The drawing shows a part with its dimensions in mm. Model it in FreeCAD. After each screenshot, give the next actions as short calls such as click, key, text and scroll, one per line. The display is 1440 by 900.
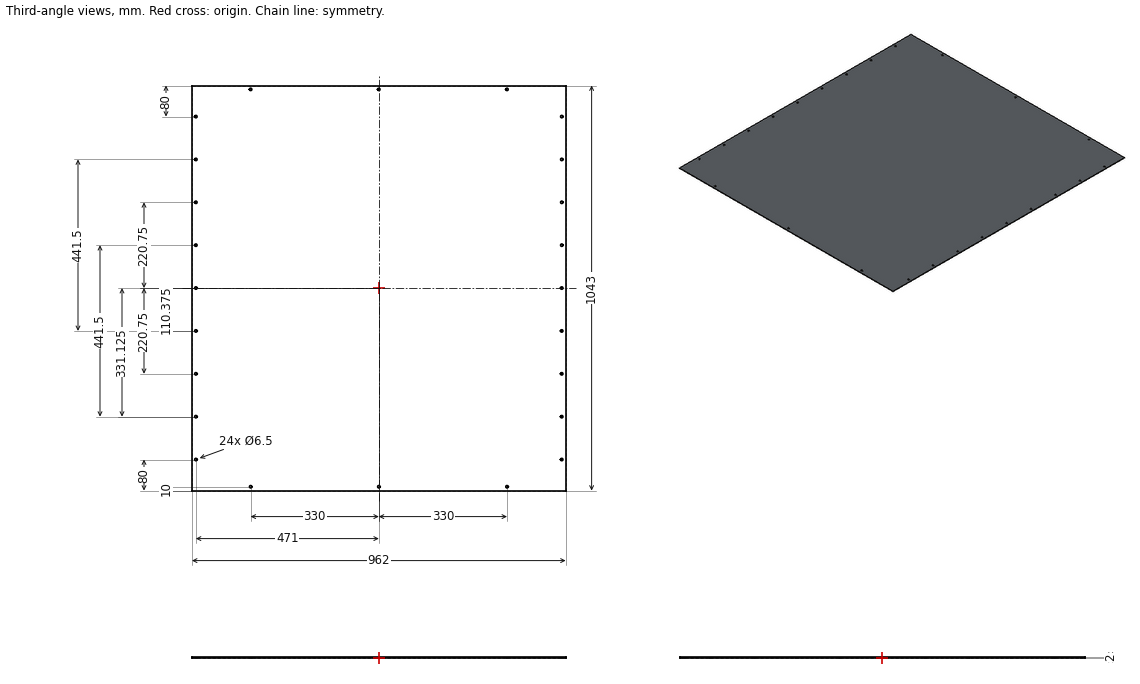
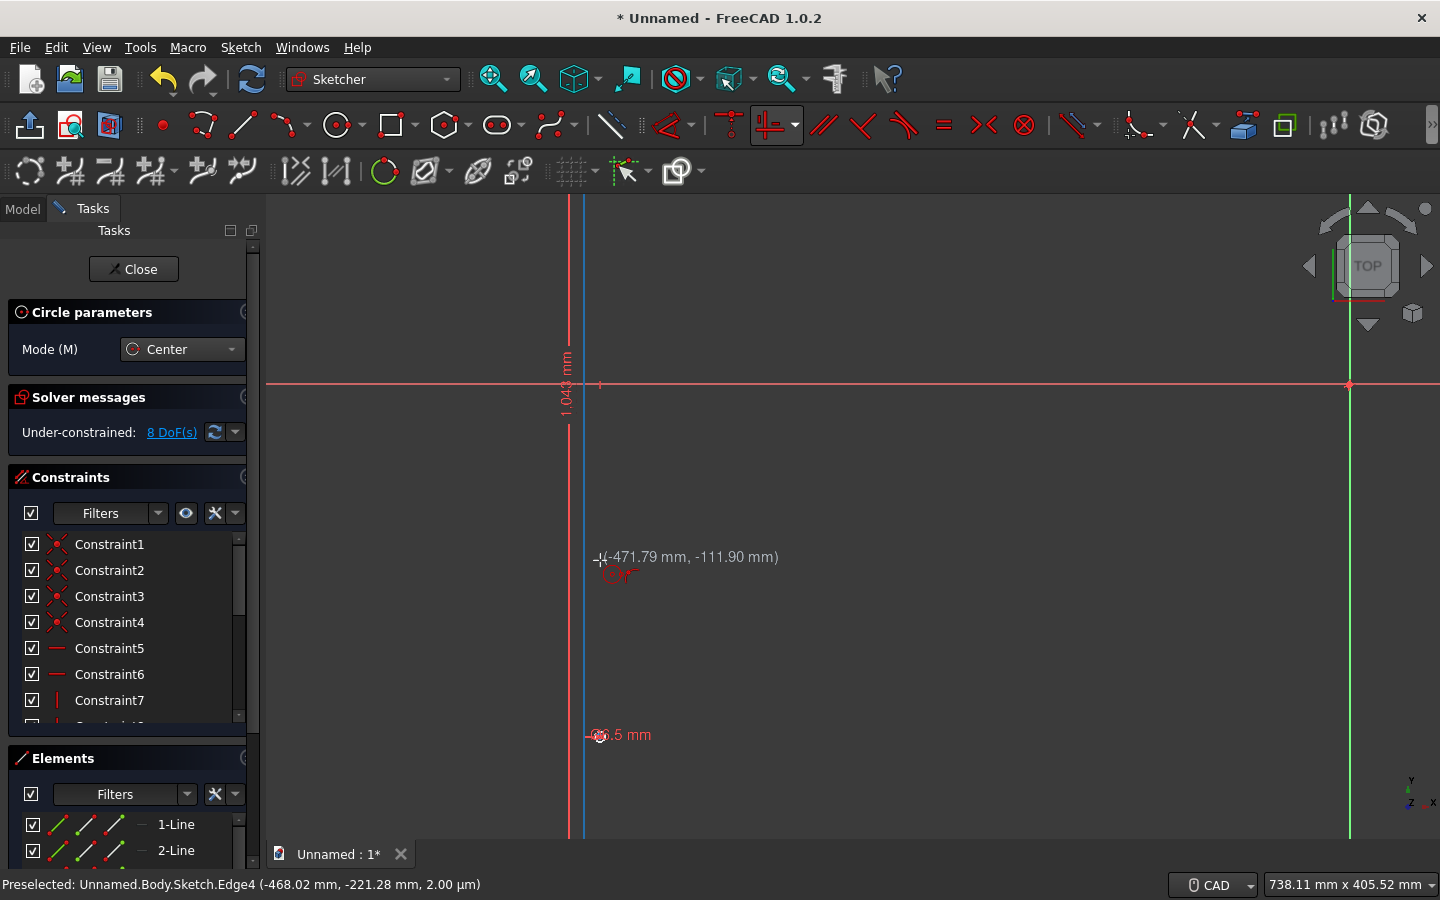
click(600, 560)
move(604, 556)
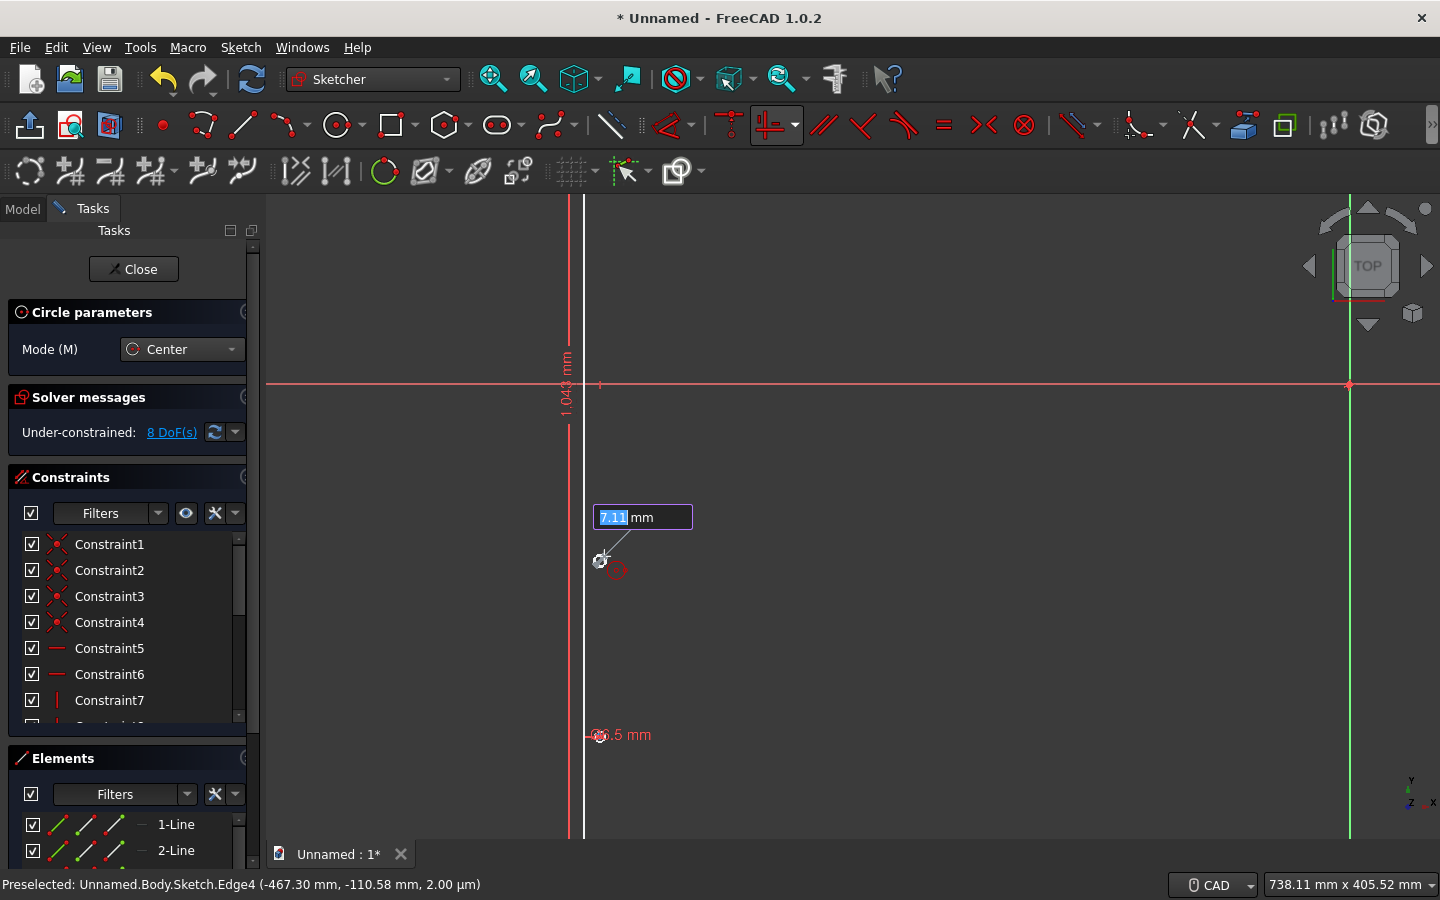
text(6.5)
key(Return)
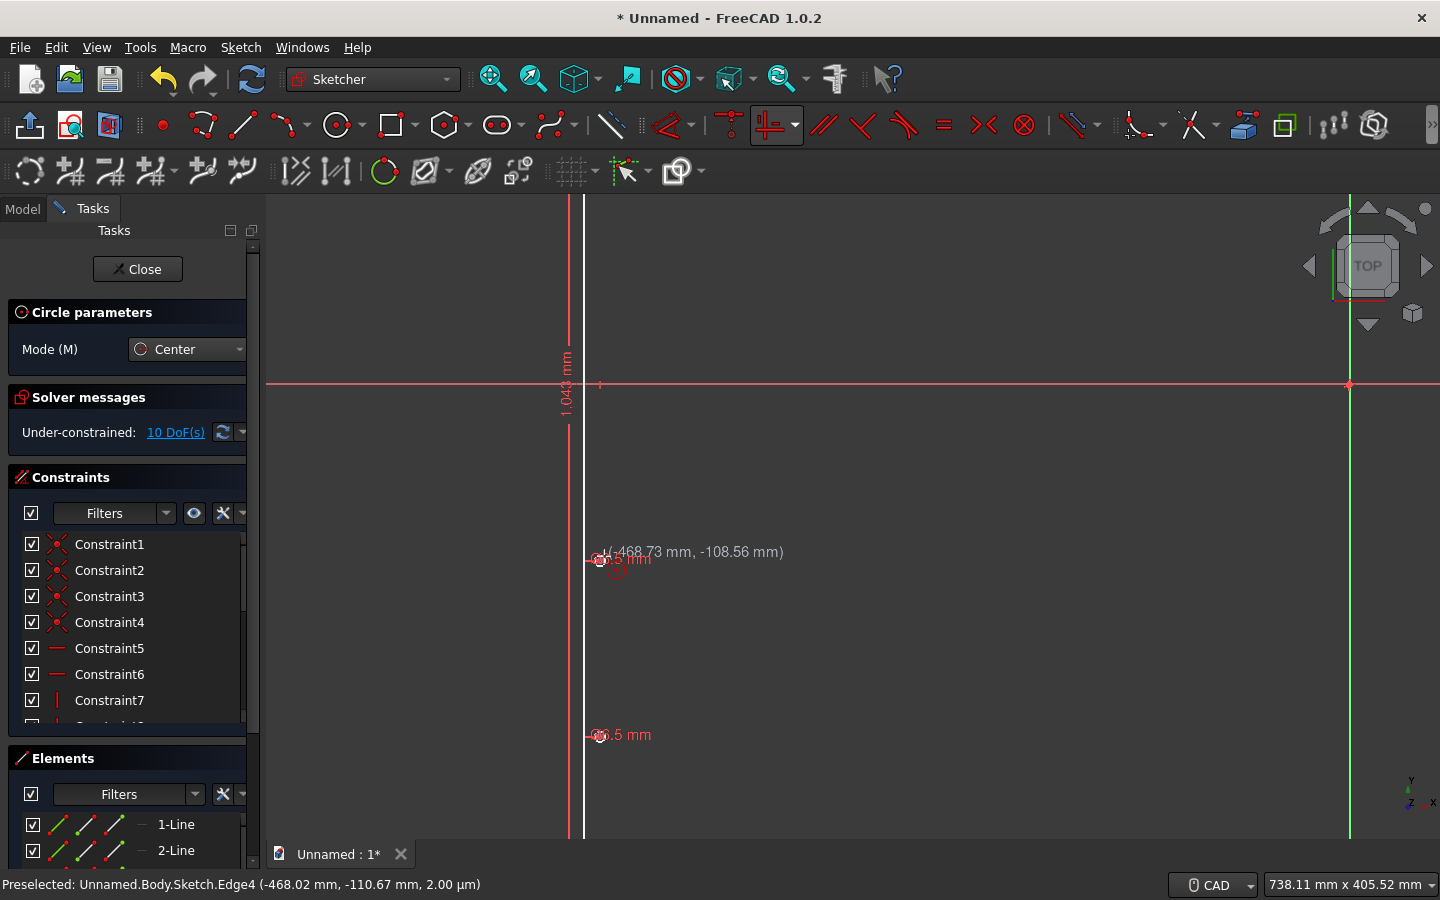
scroll(600, 560, down, 7)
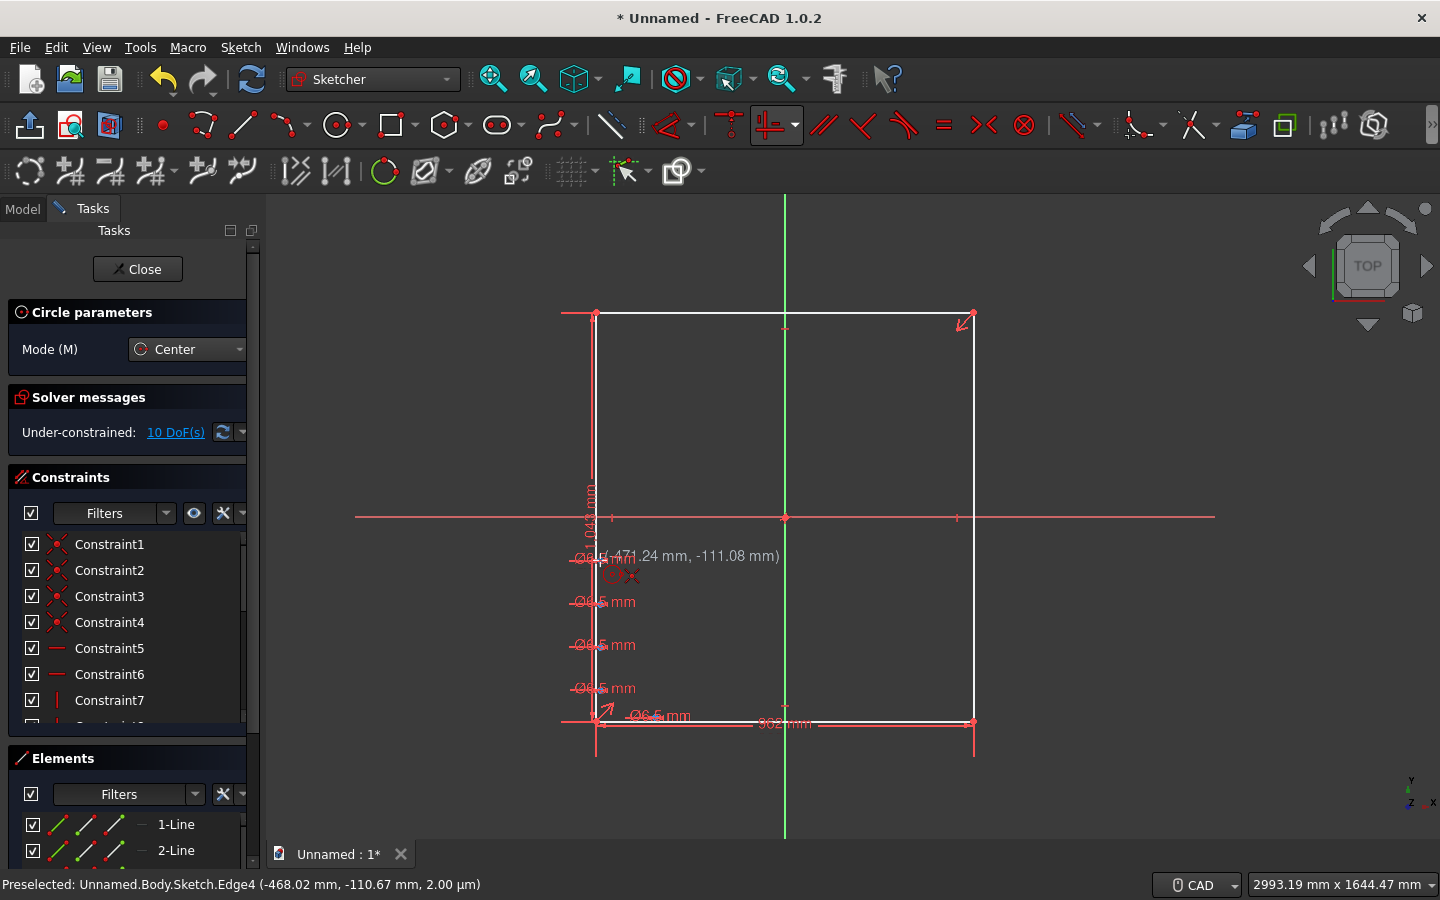
scroll(785, 718, up, 15)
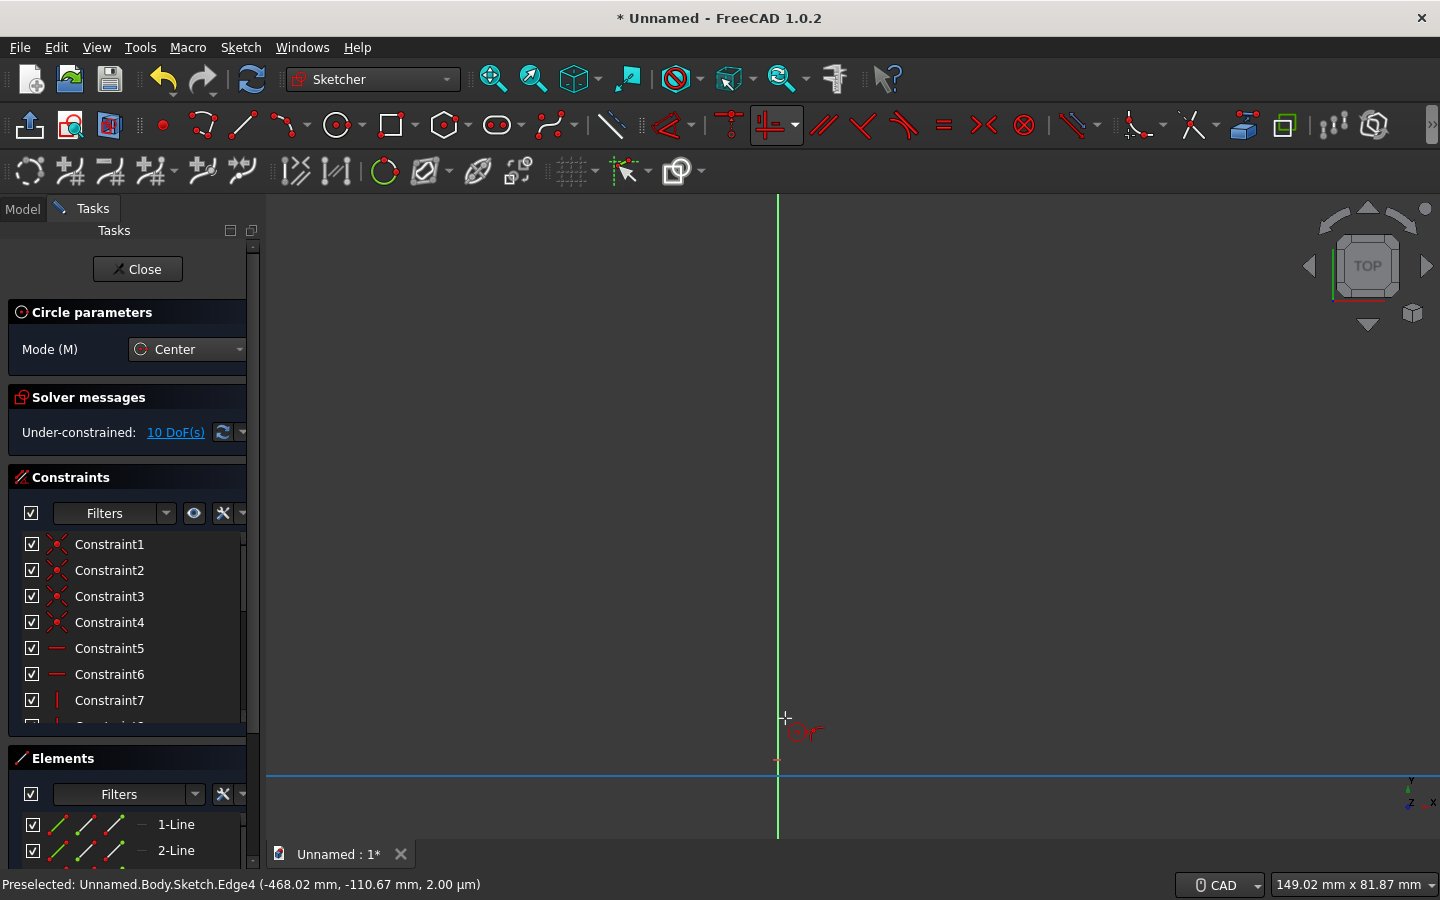
scroll(785, 718, down, 15)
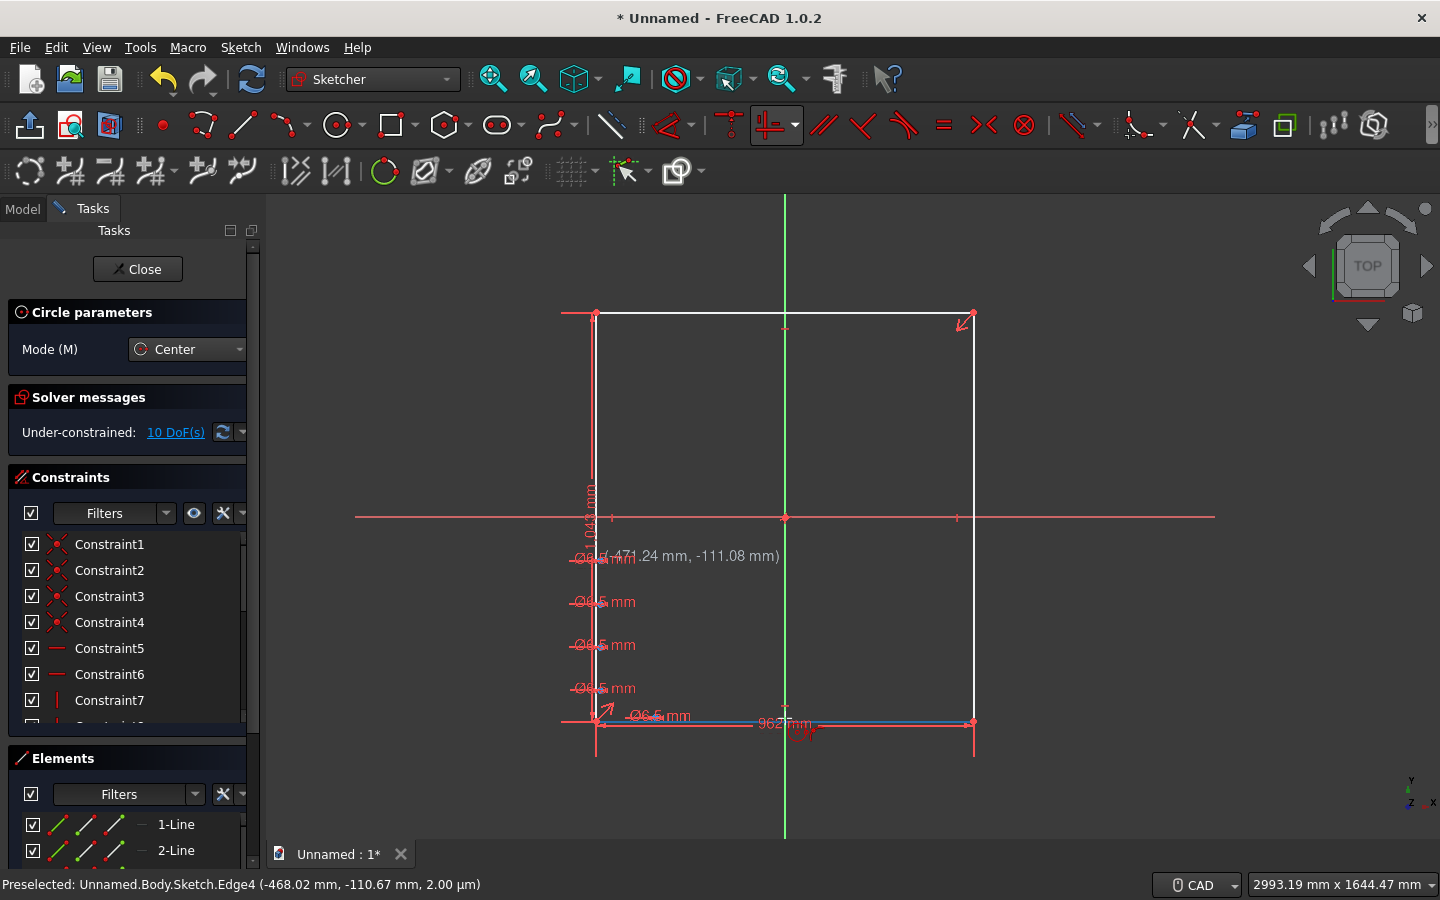
scroll(785, 718, up, 7)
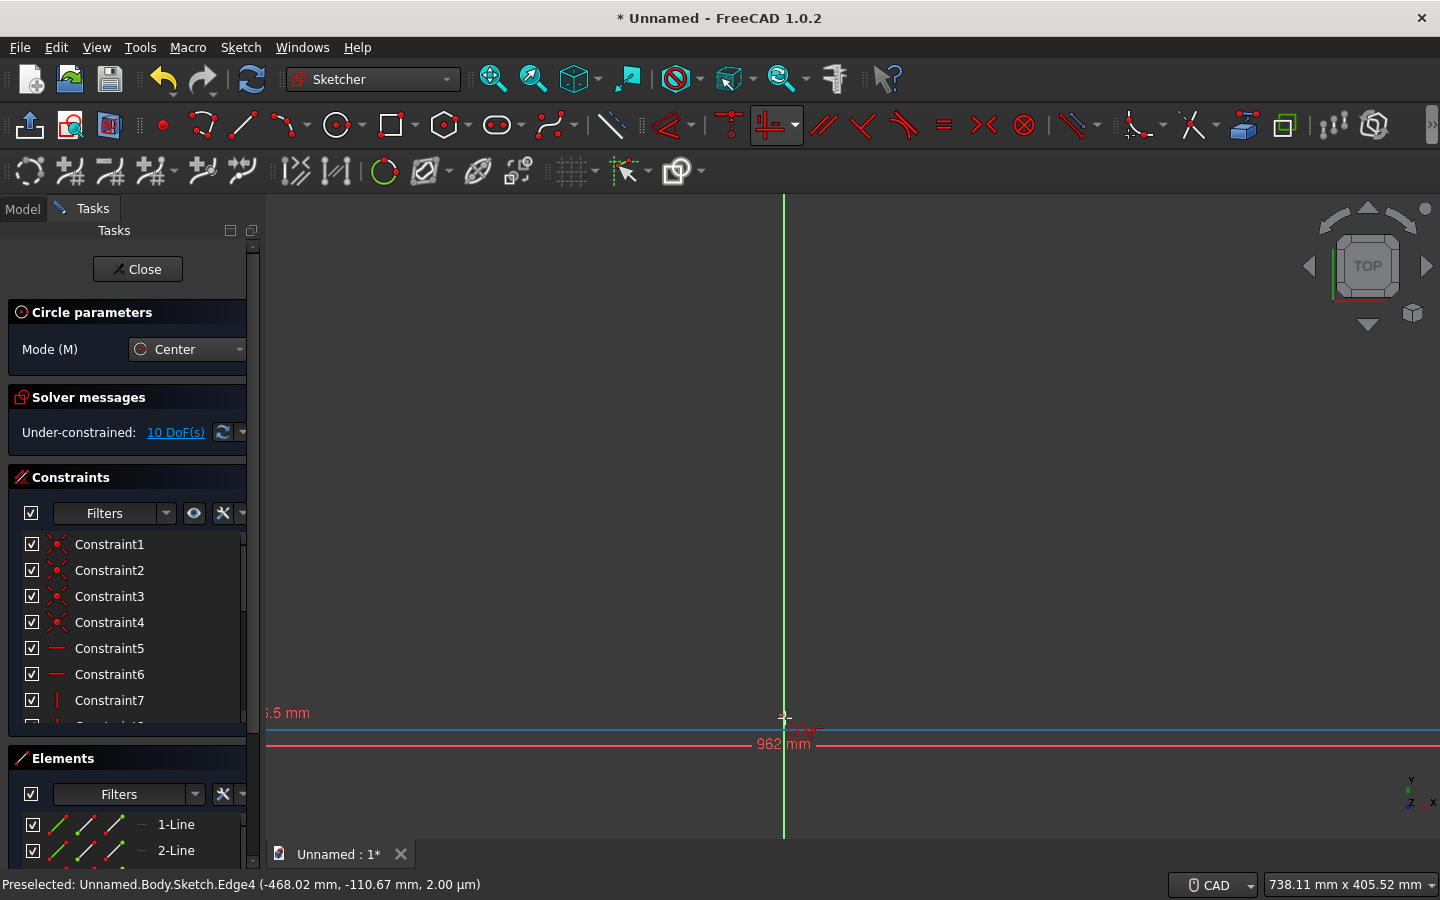
click(784, 714)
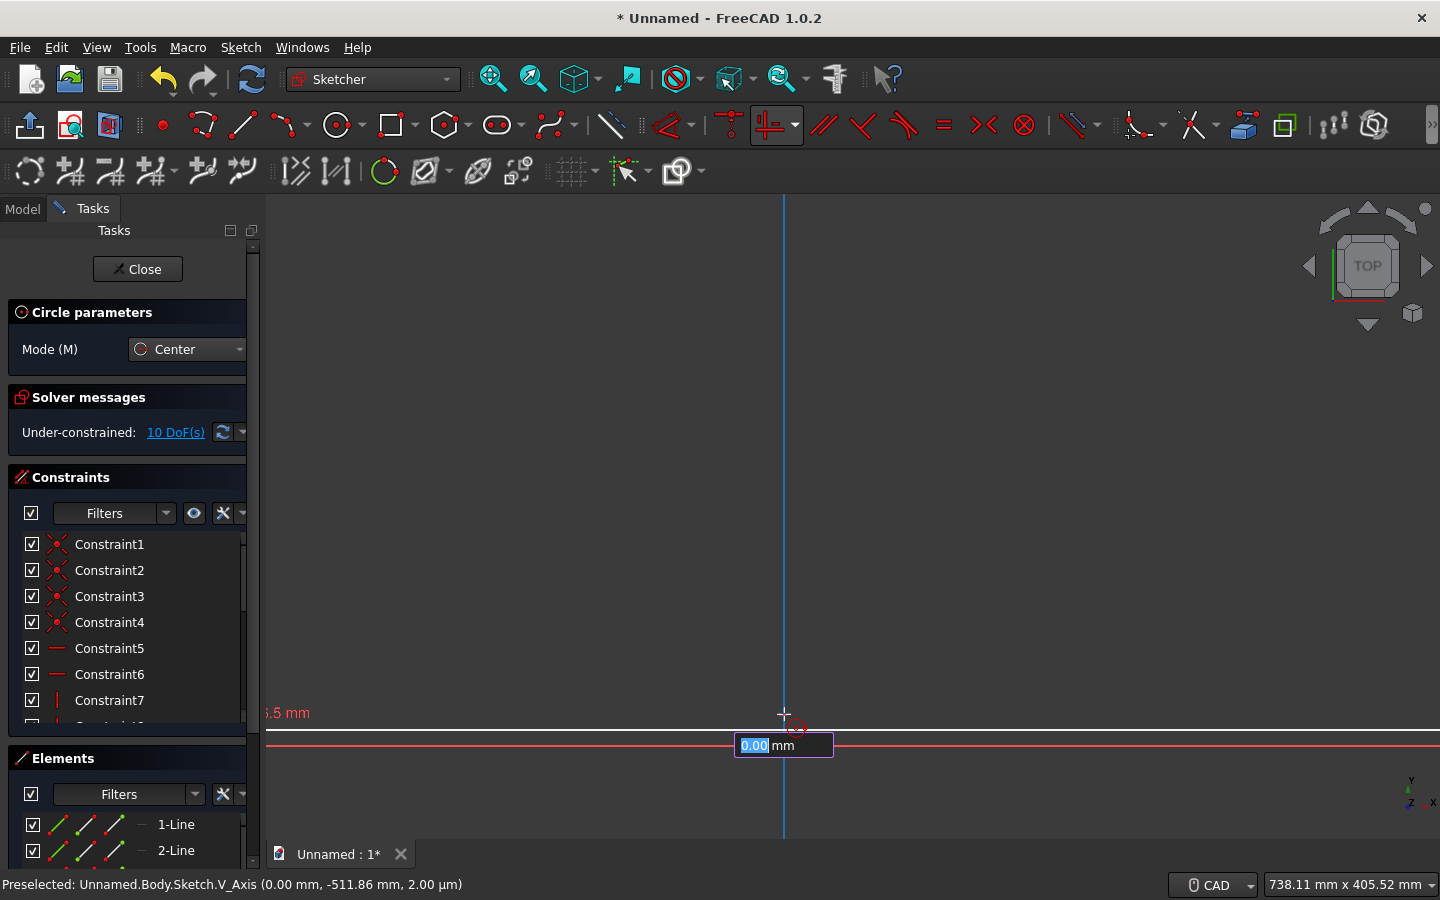
scroll(789, 713, up, 6)
move(787, 710)